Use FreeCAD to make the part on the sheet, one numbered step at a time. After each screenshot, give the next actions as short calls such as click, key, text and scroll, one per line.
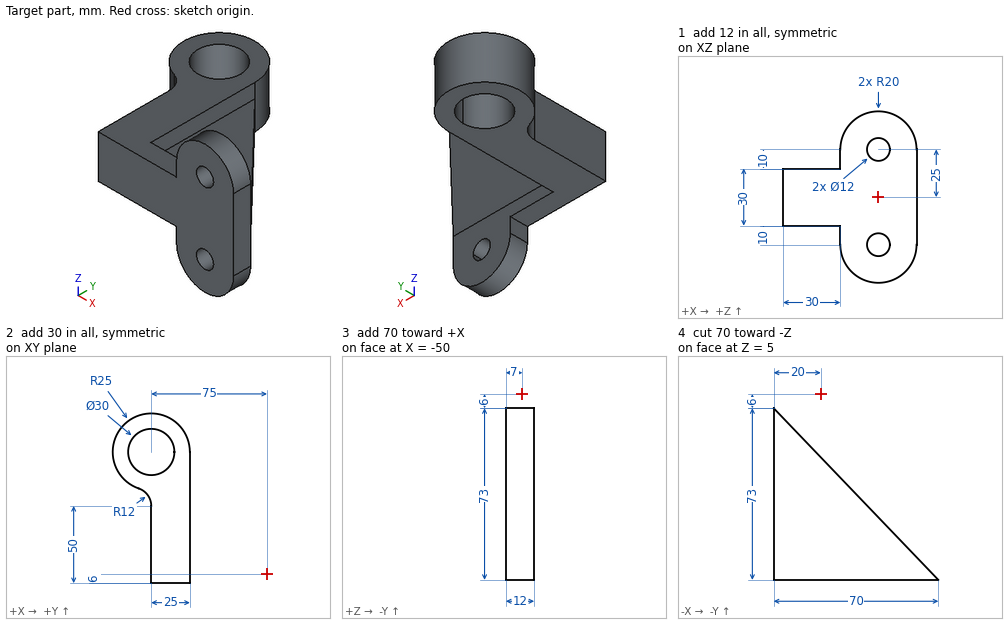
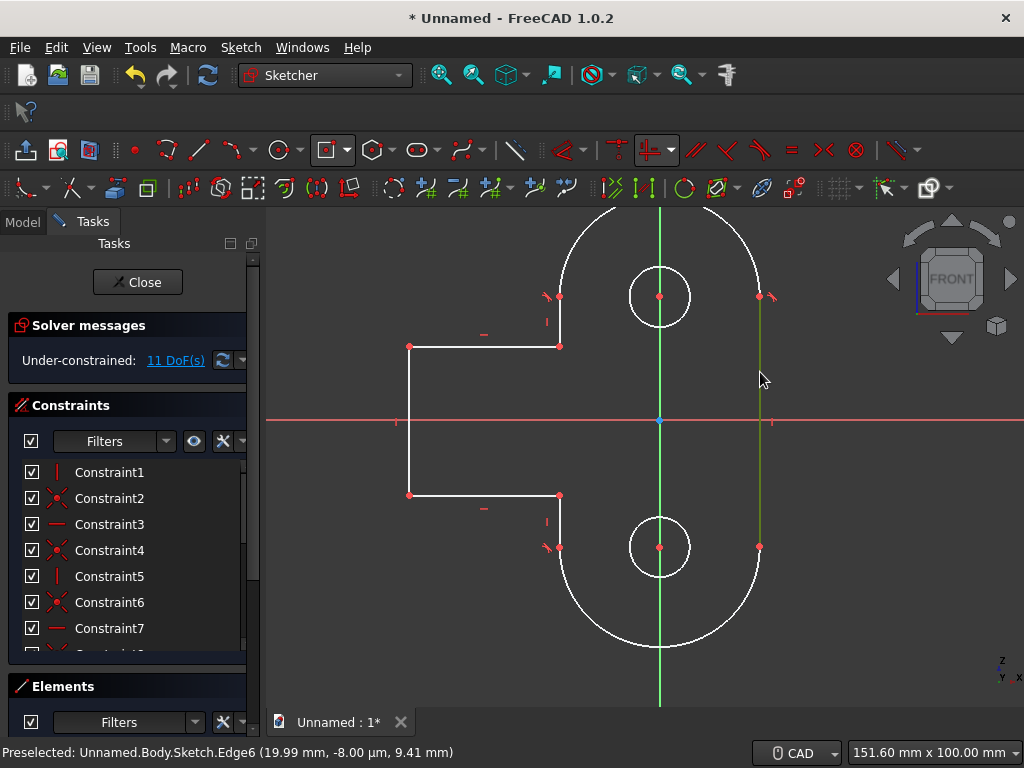
click(601, 628)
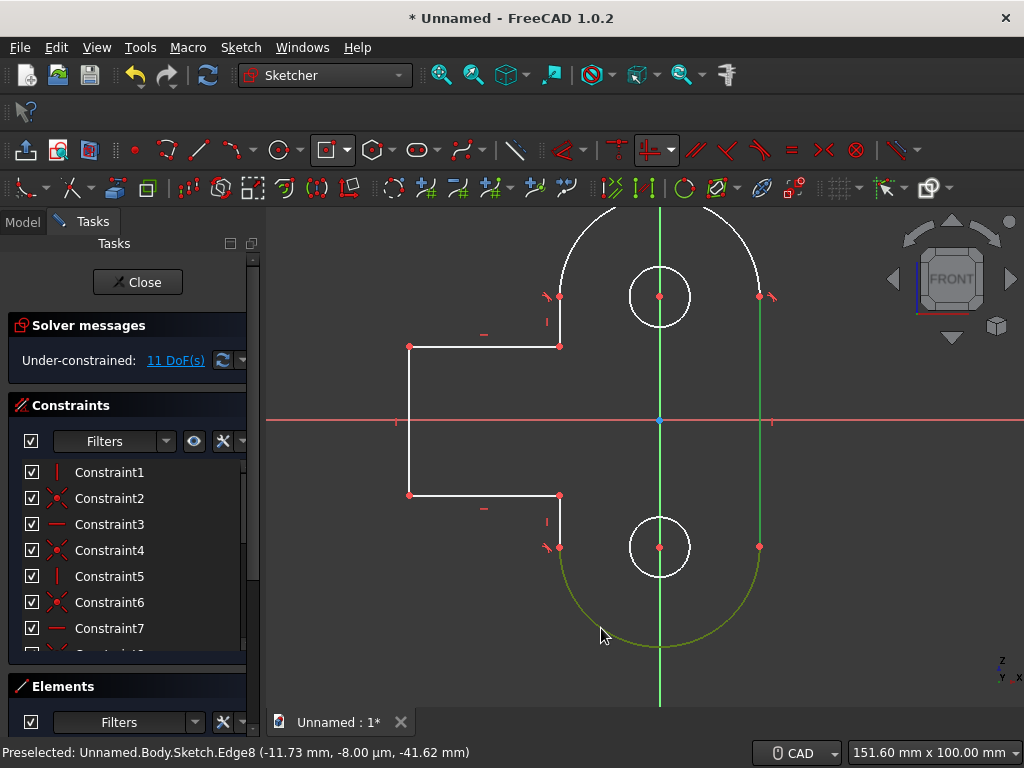
click(760, 150)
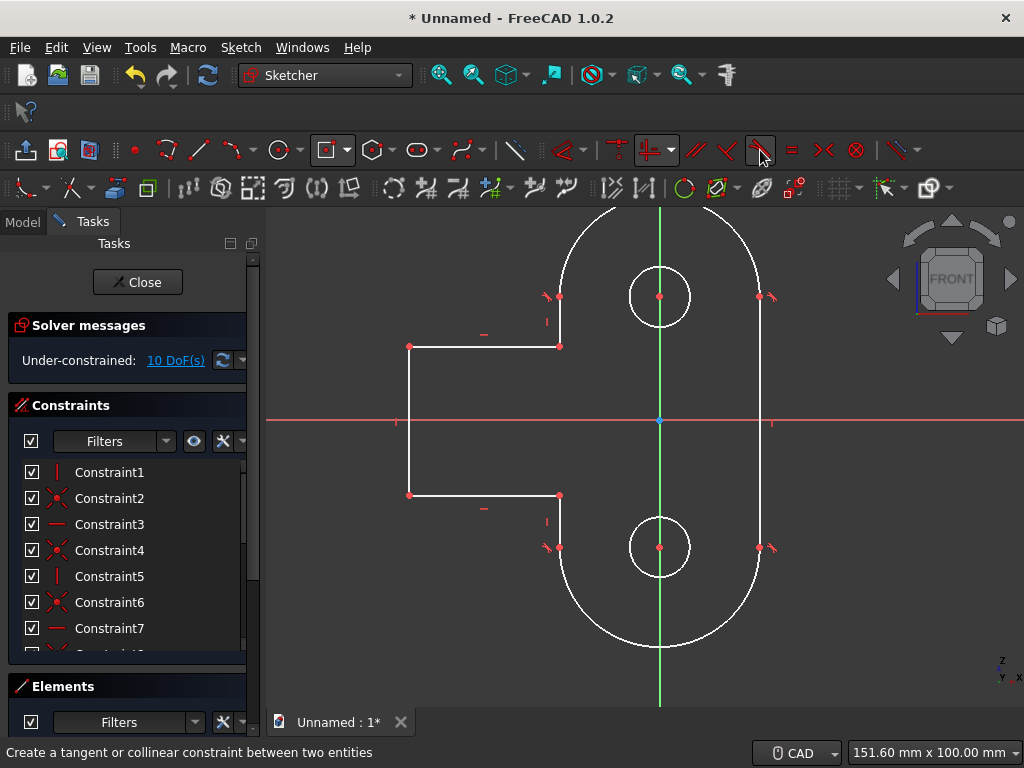
click(741, 238)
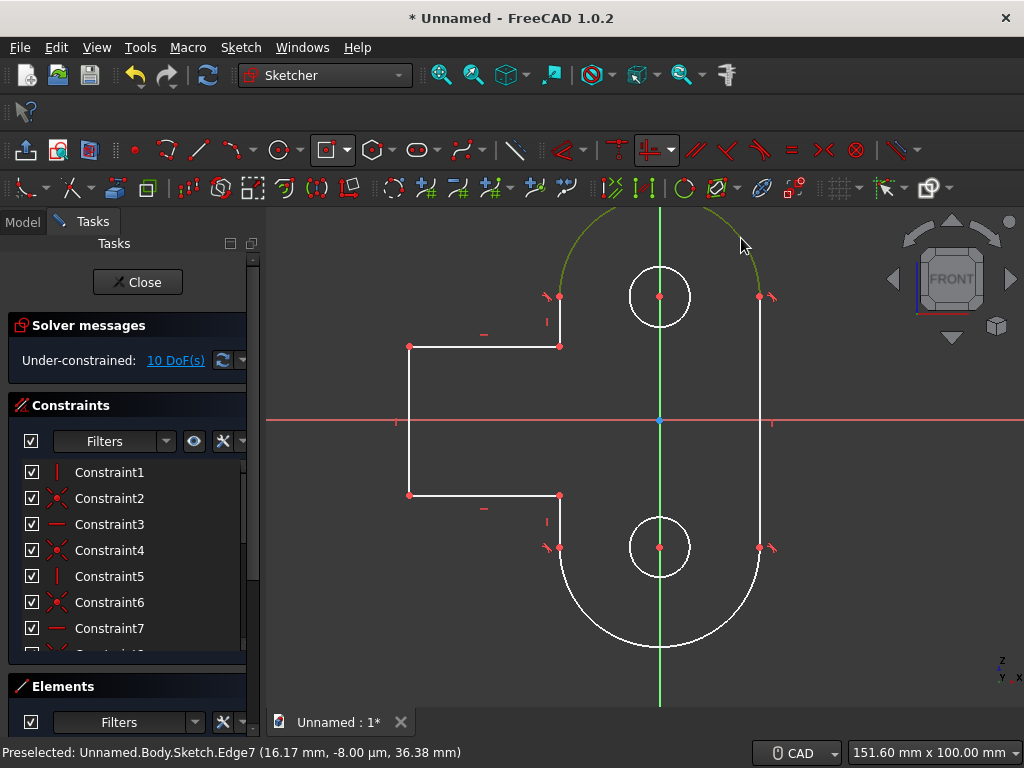
click(601, 628)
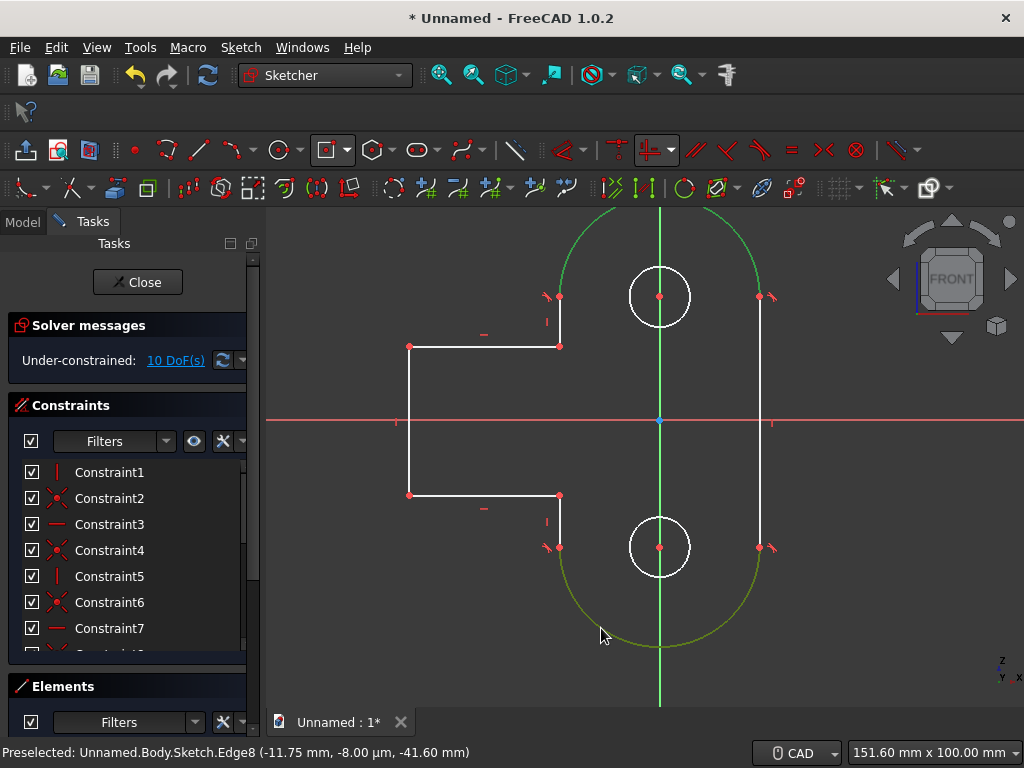
click(792, 150)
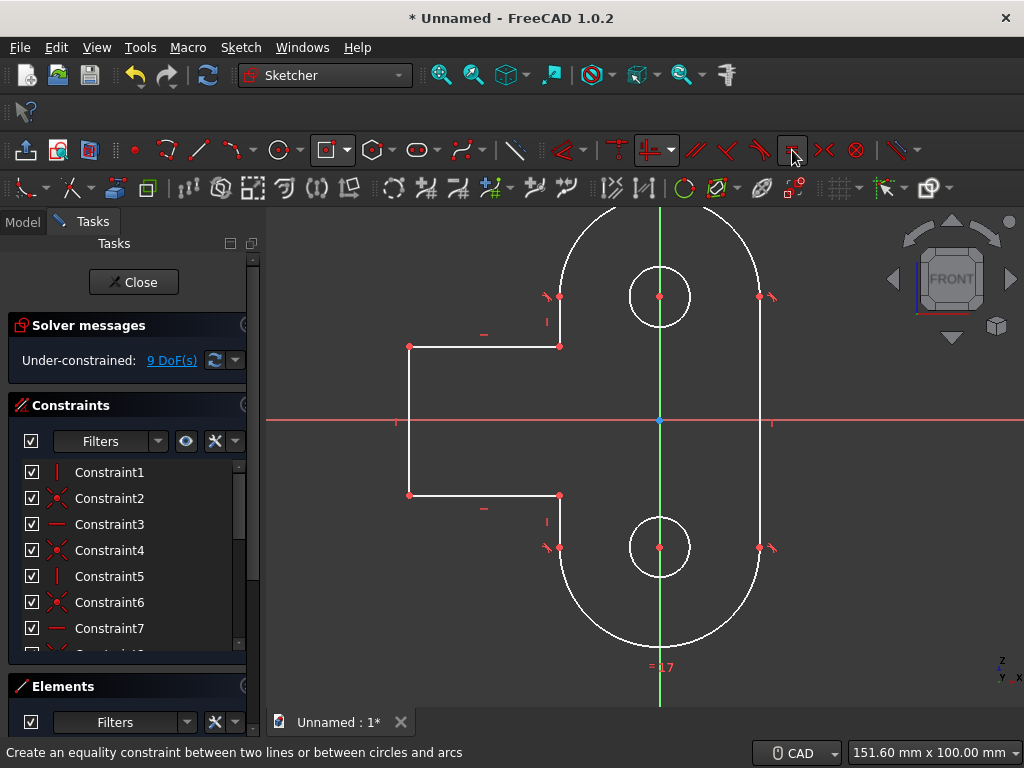
click(681, 275)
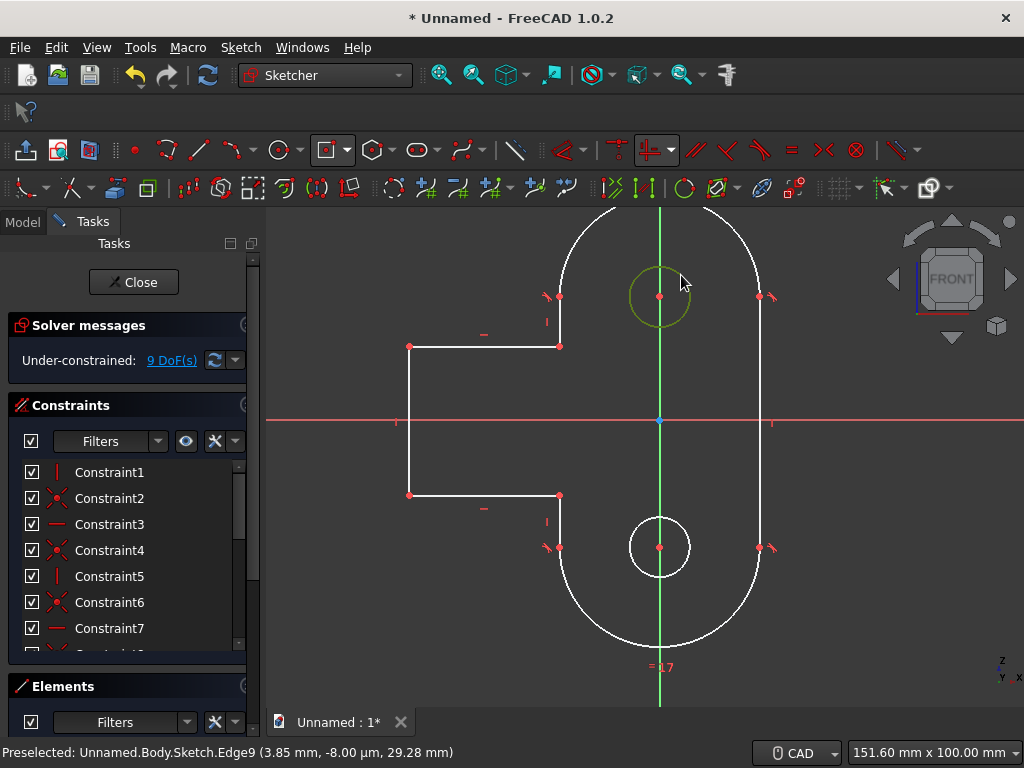
click(681, 526)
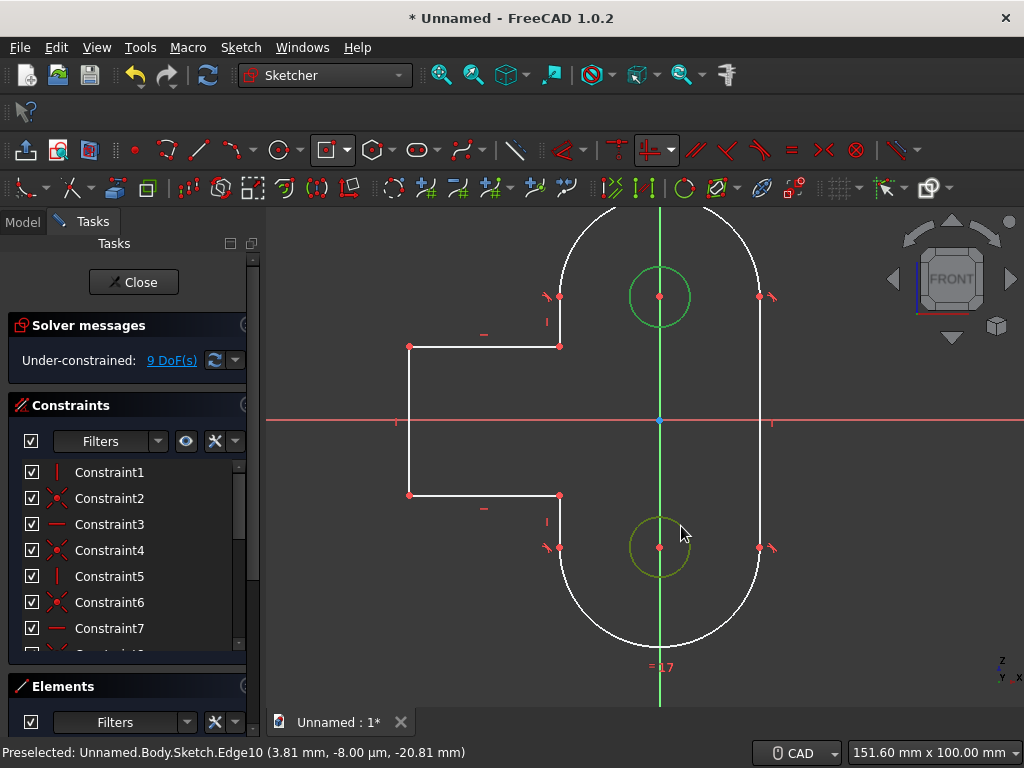
click(792, 150)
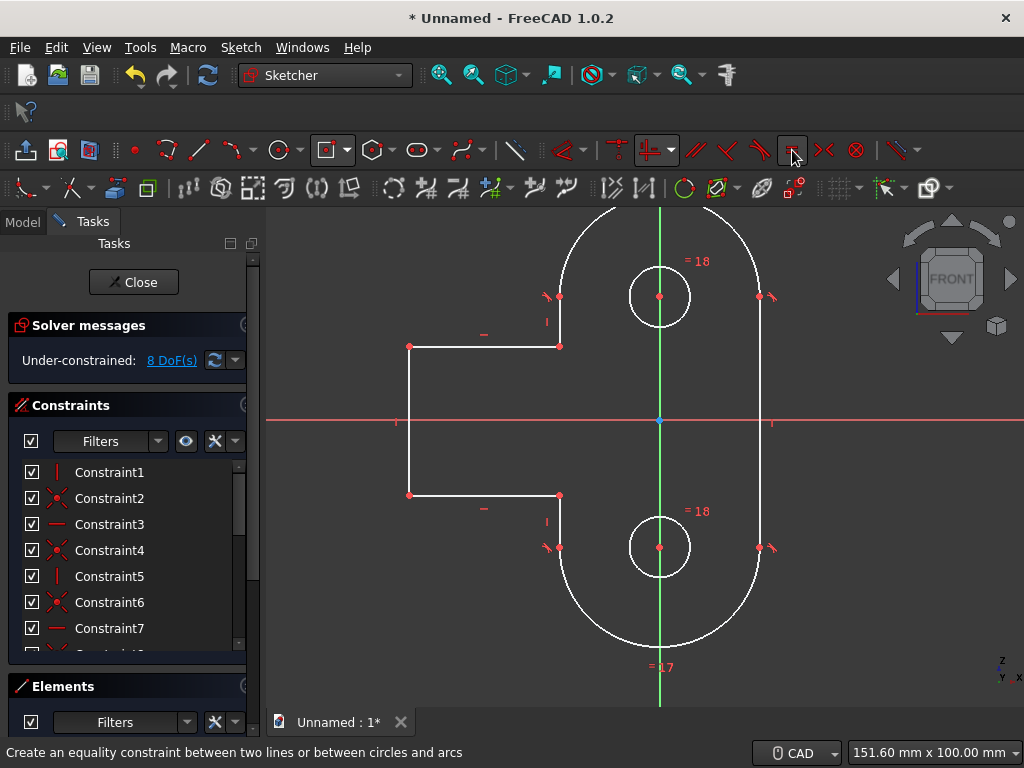
click(660, 297)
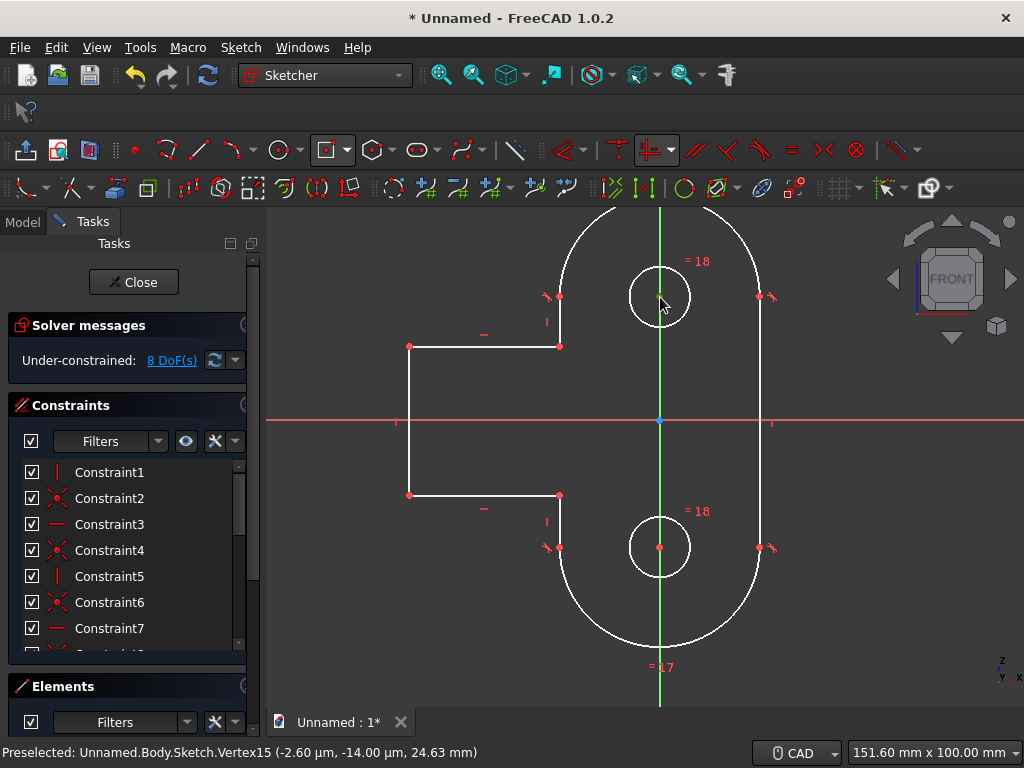
click(660, 616)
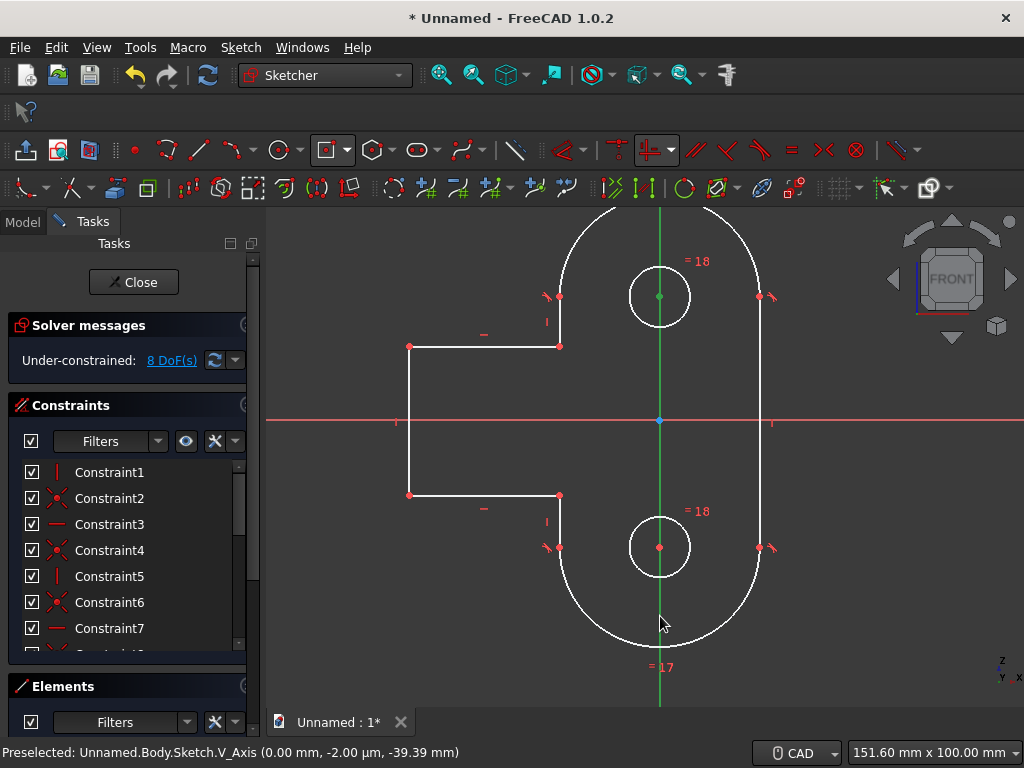
click(618, 150)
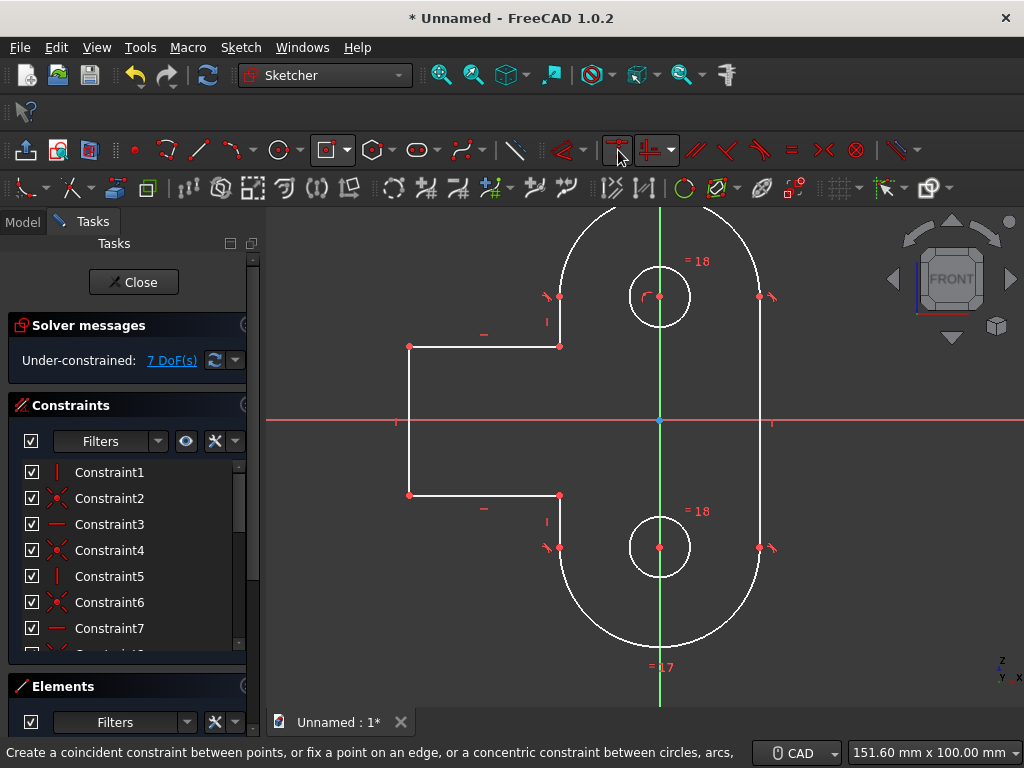
click(562, 150)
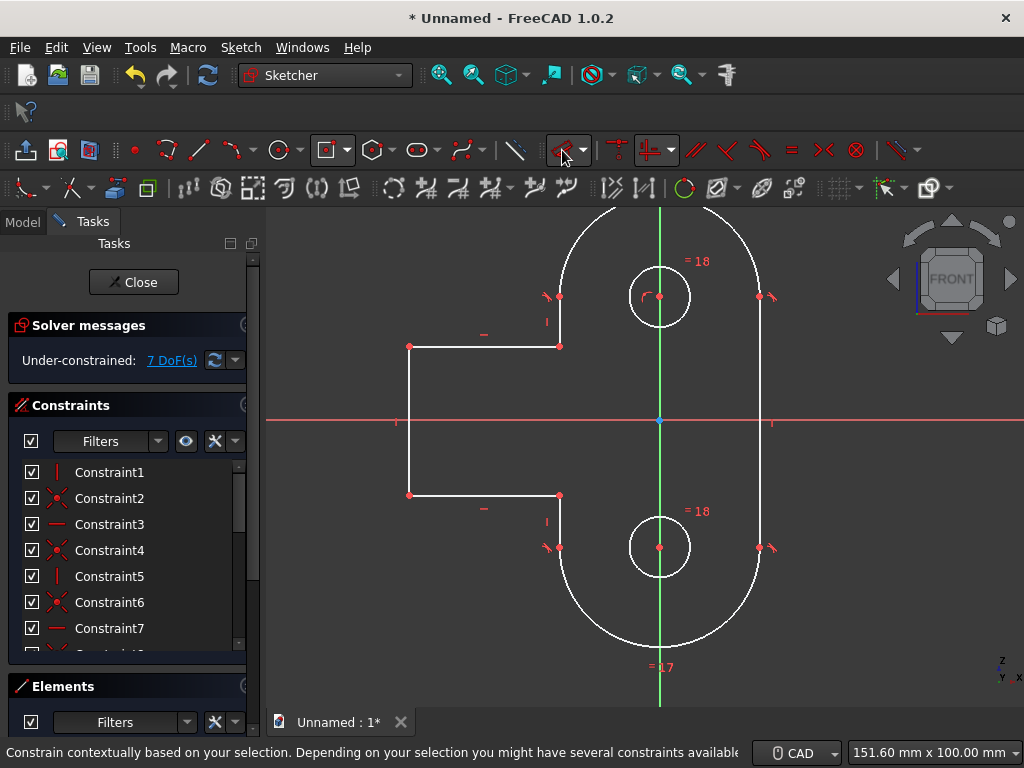
click(741, 238)
click(791, 280)